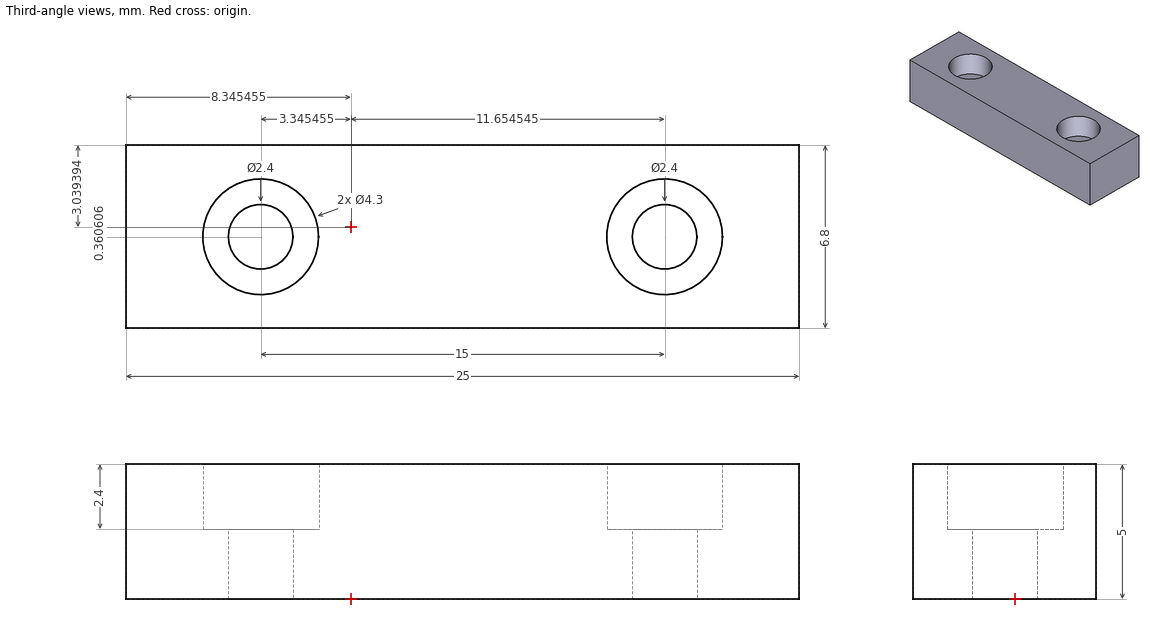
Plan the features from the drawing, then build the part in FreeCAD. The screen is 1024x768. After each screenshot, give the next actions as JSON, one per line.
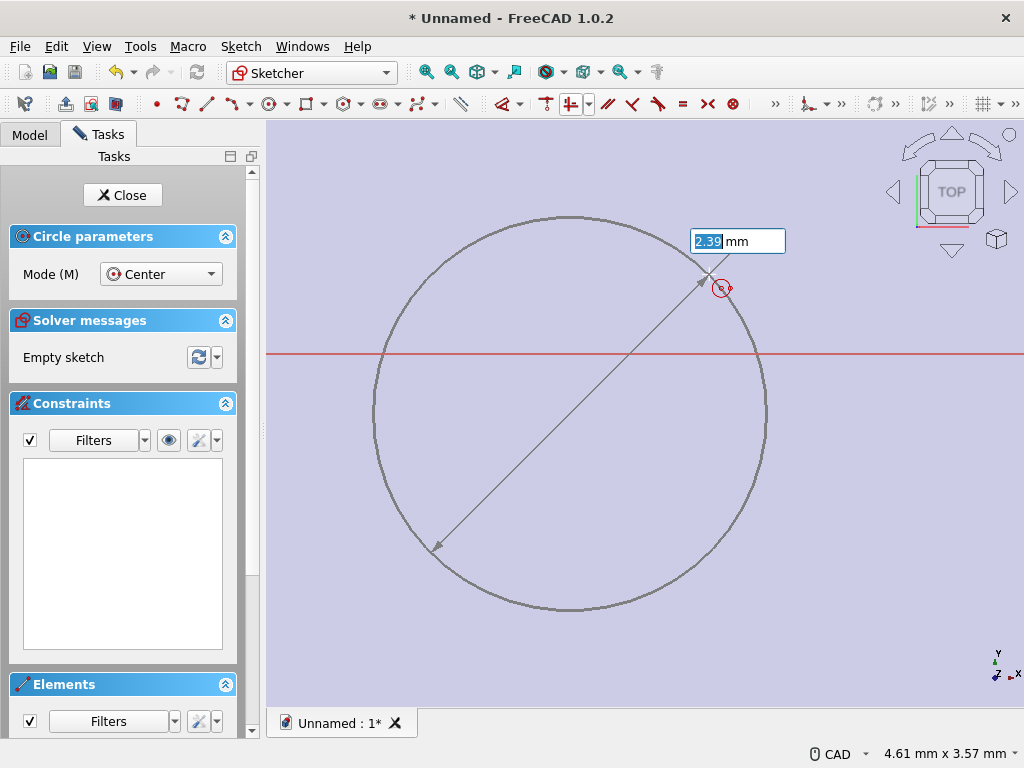
{"action": "type", "text": "2.4"}
{"action": "key", "text": "Return"}
{"action": "key", "text": "Escape"}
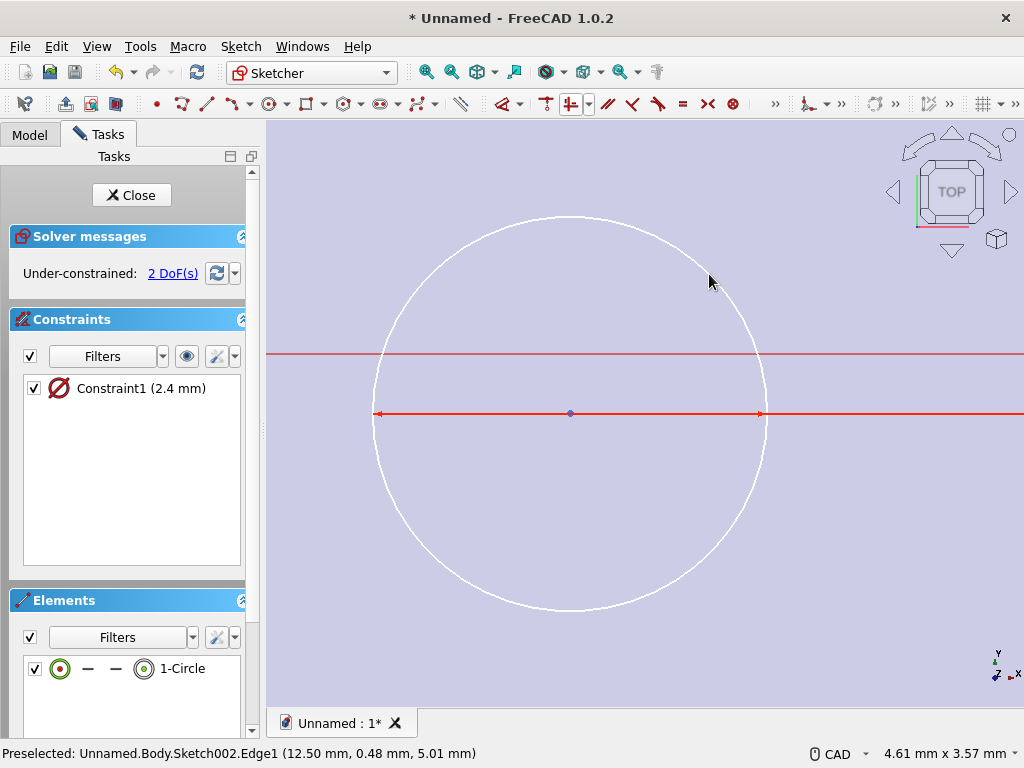
{"action": "left_click", "coordinate": [502, 104]}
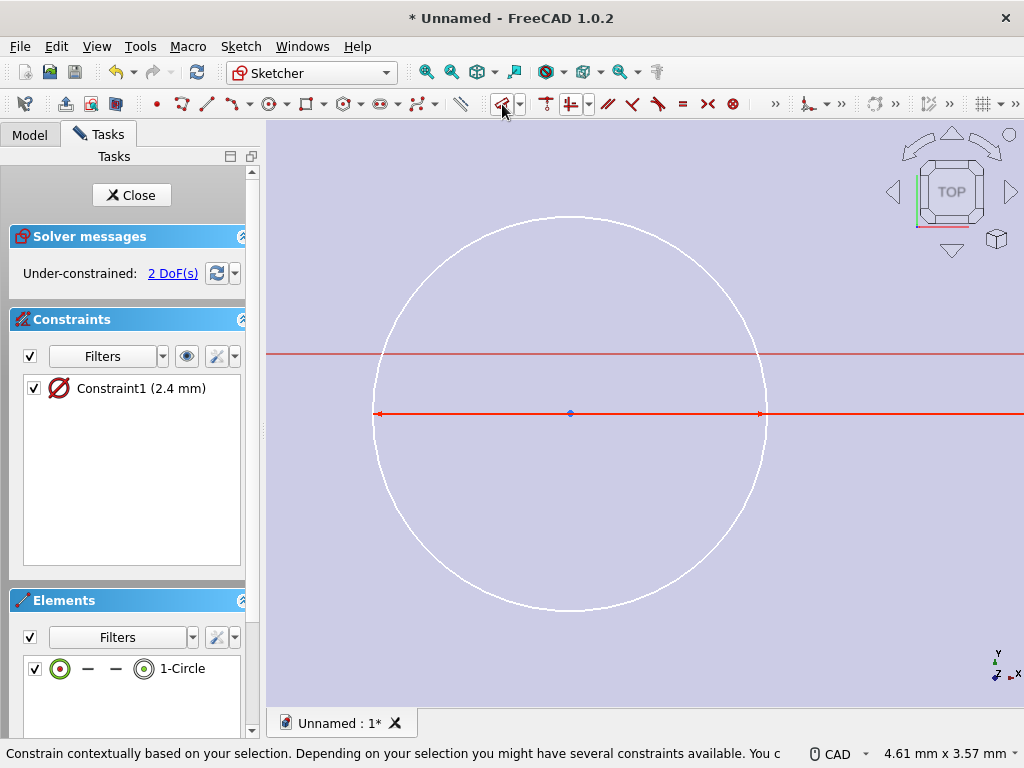
{"action": "left_click", "coordinate": [570, 414]}
{"action": "left_click", "coordinate": [604, 384]}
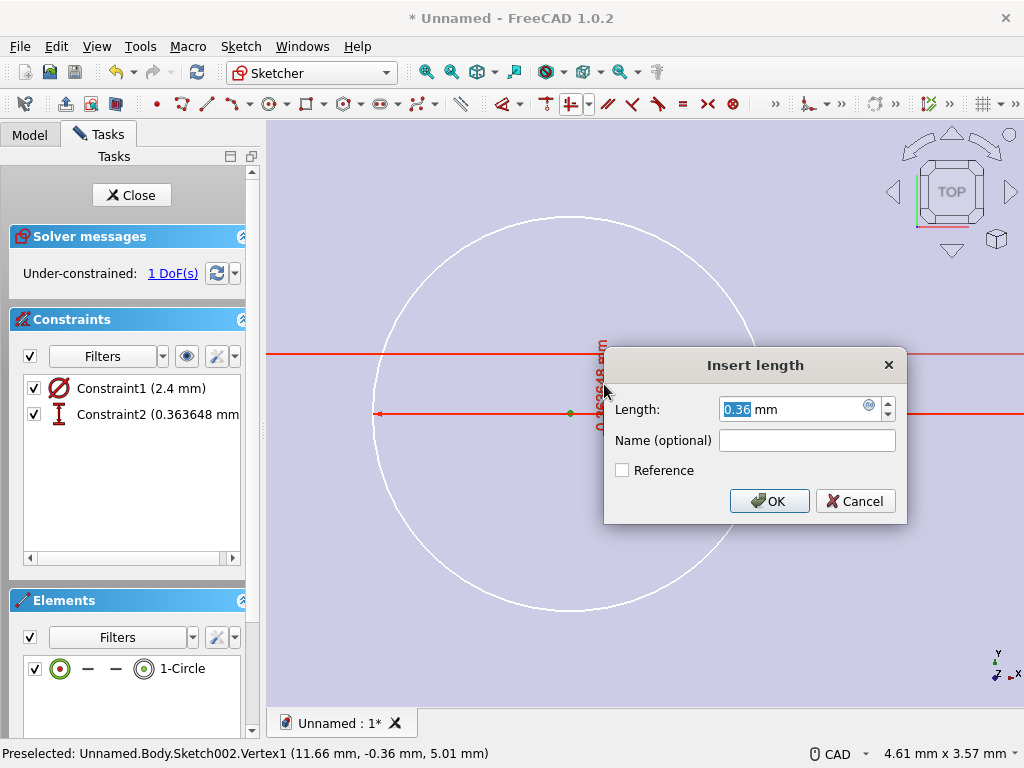
{"action": "type", "text": "0.360606"}
{"action": "key", "text": "Return"}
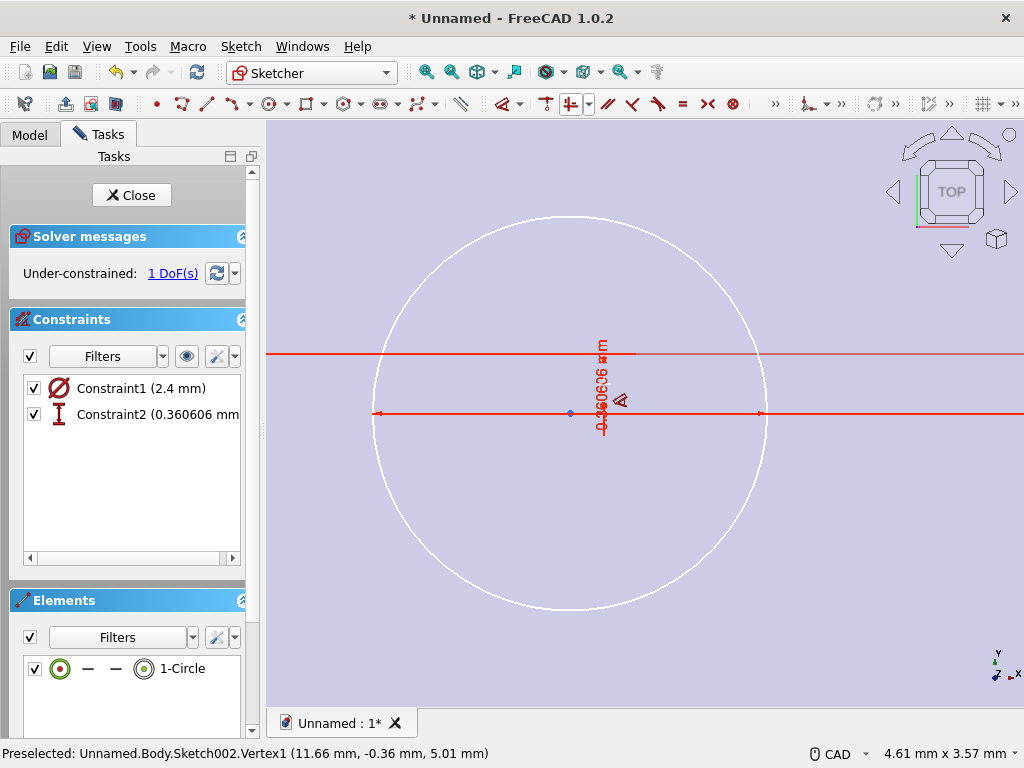
{"action": "left_click", "coordinate": [570, 413]}
{"action": "left_click", "coordinate": [432, 320]}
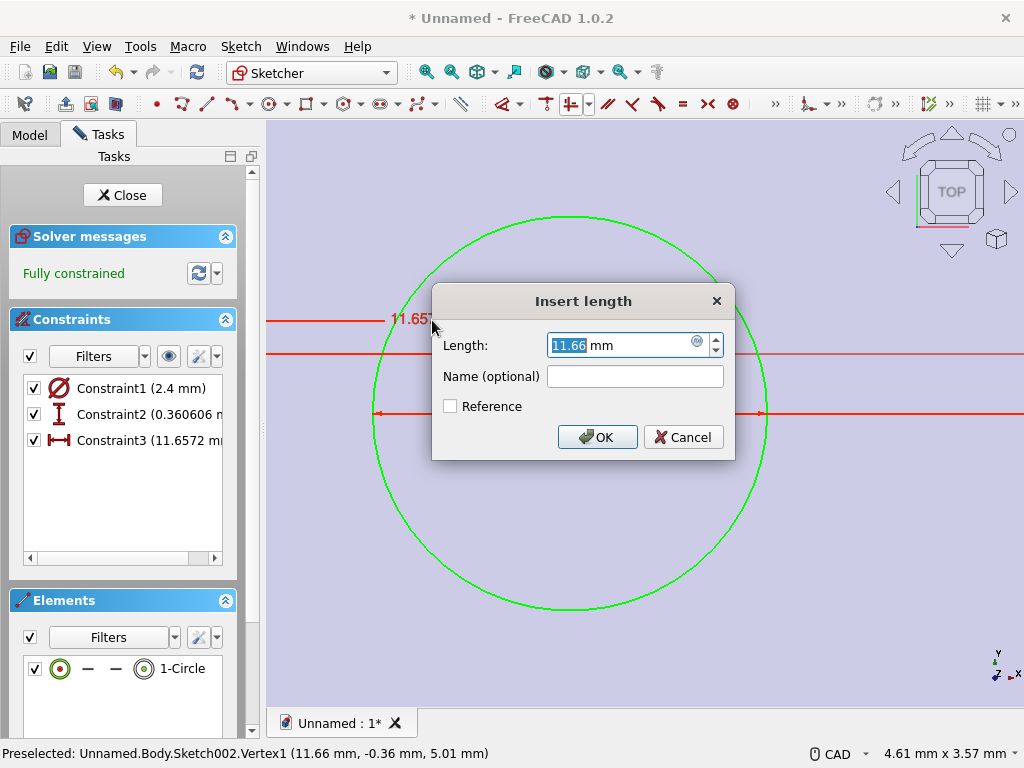
{"action": "type", "text": "11.654545"}
{"action": "key", "text": "Return"}
{"action": "key", "text": "Escape"}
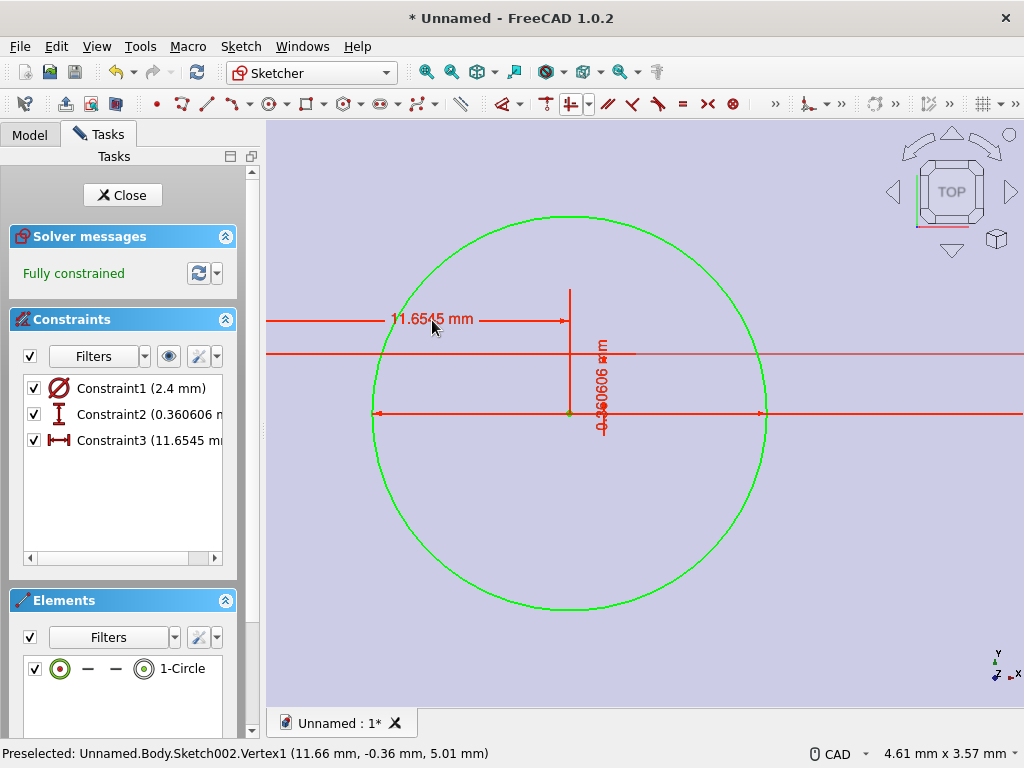
{"action": "left_click", "coordinate": [123, 195]}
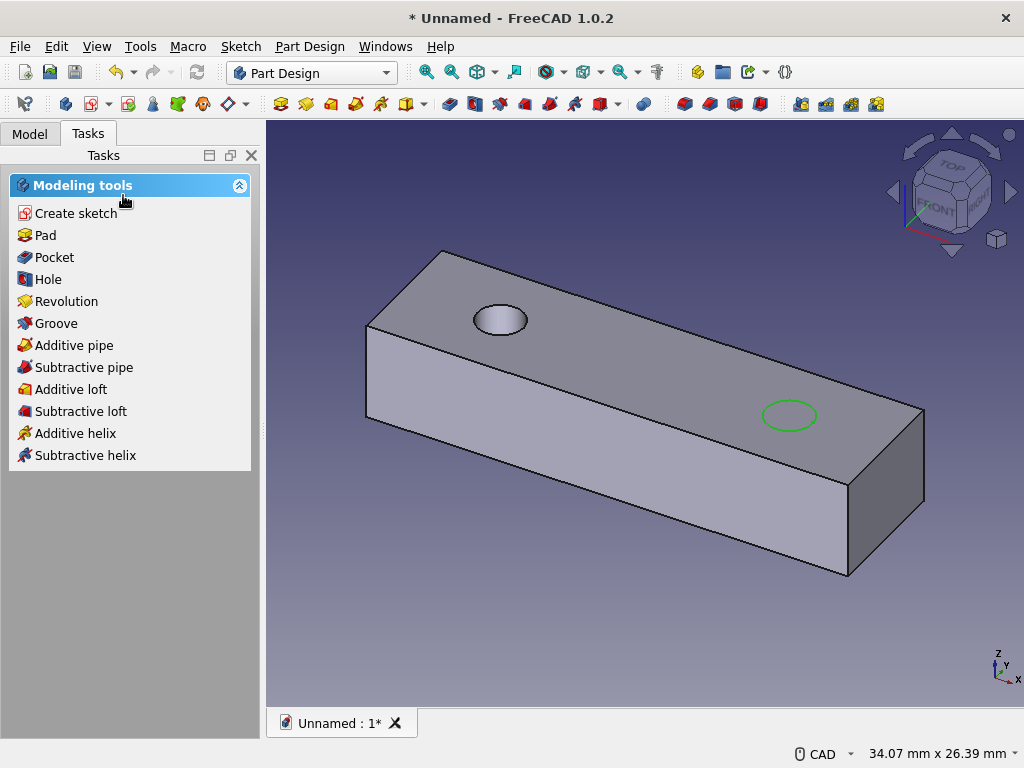
{"action": "left_click", "coordinate": [450, 104]}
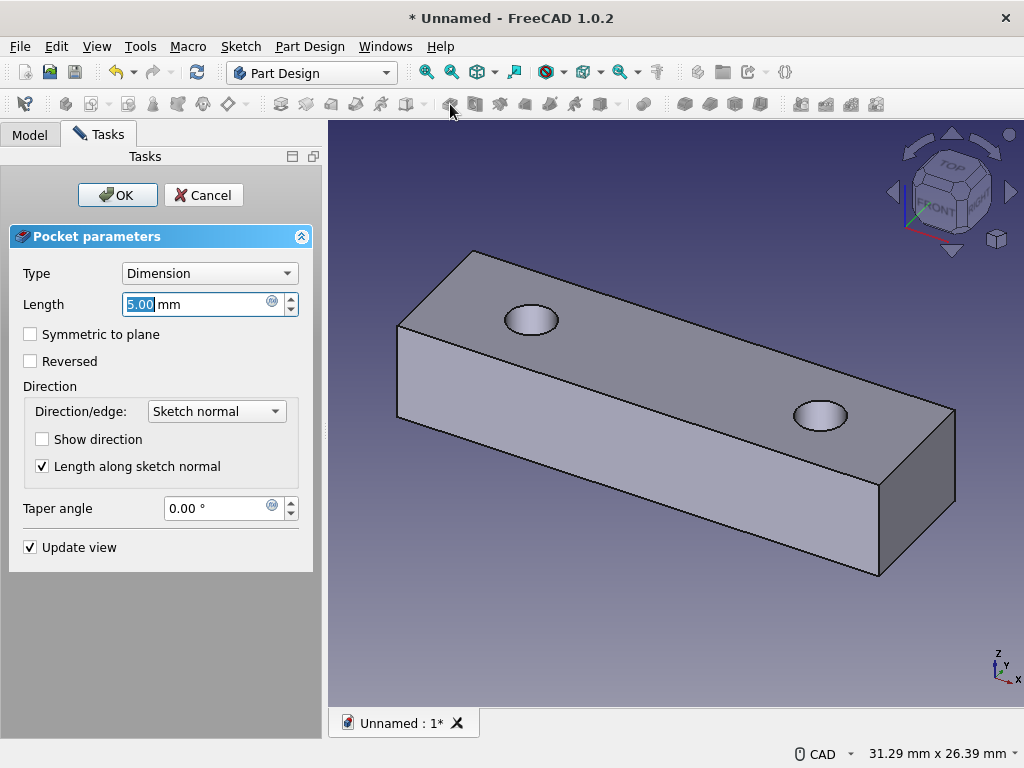
{"action": "left_click", "coordinate": [210, 274]}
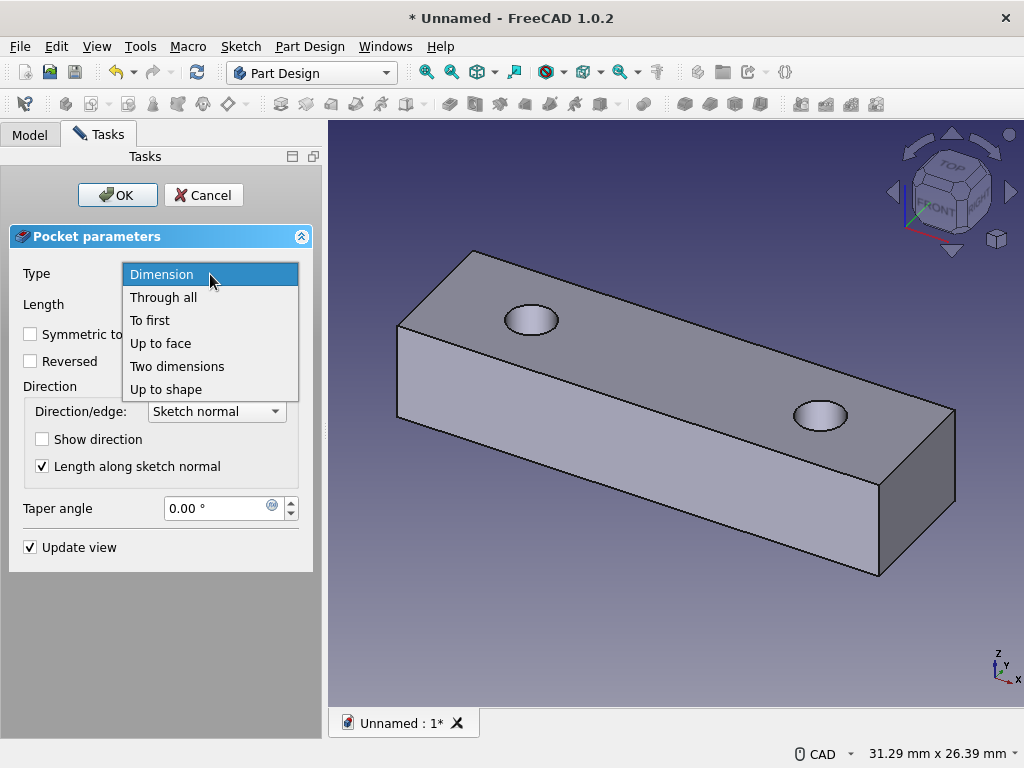
{"action": "left_click", "coordinate": [208, 320]}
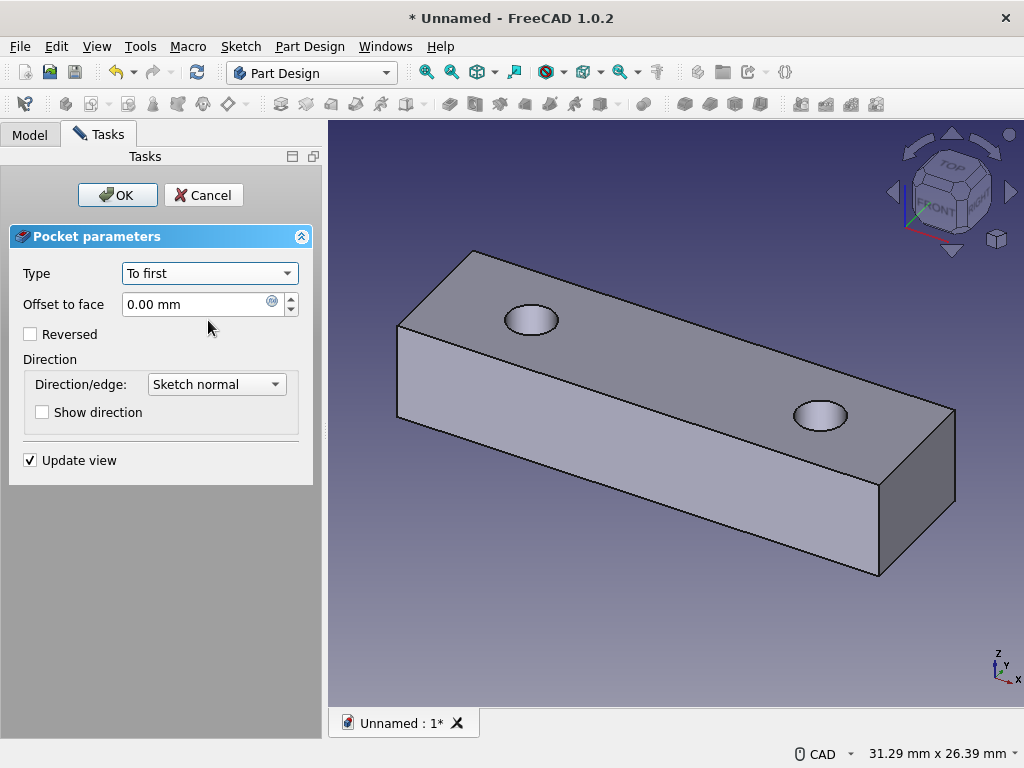
{"action": "left_click", "coordinate": [118, 195]}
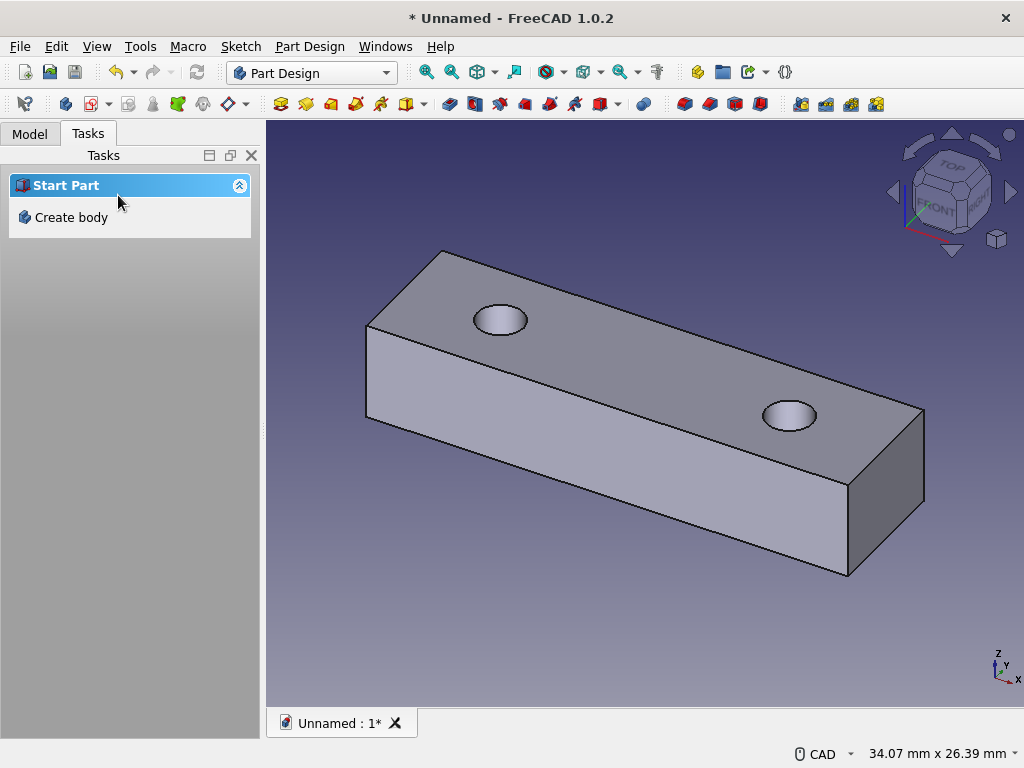
{"action": "left_click", "coordinate": [645, 367]}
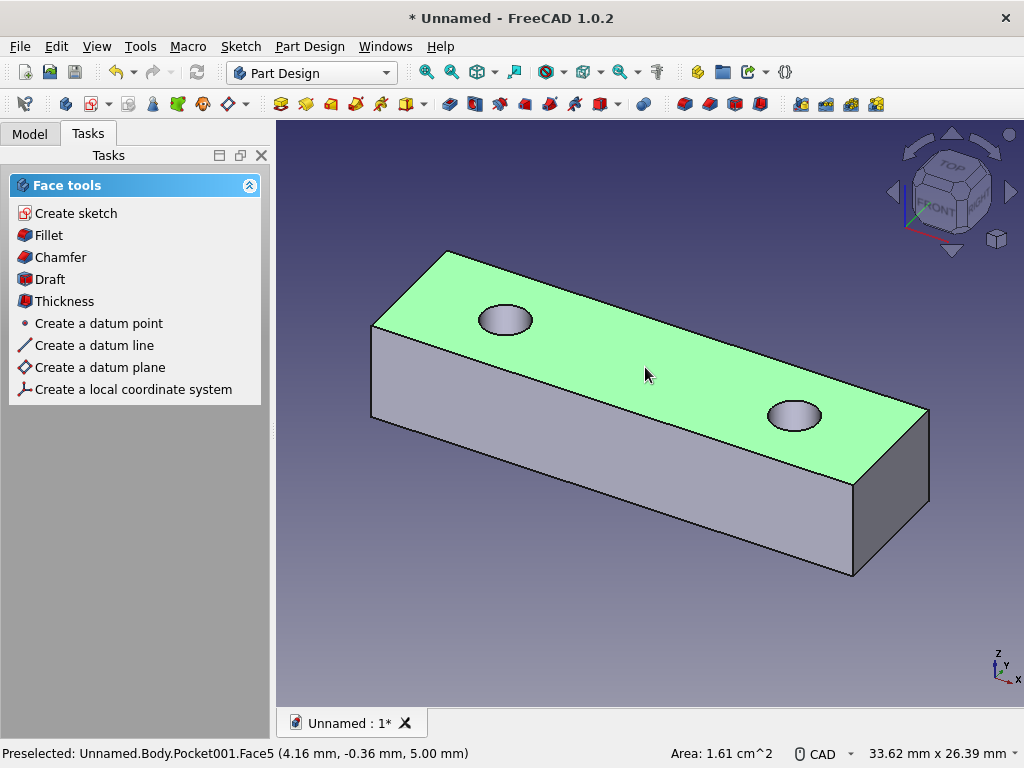
{"action": "left_click", "coordinate": [90, 104]}